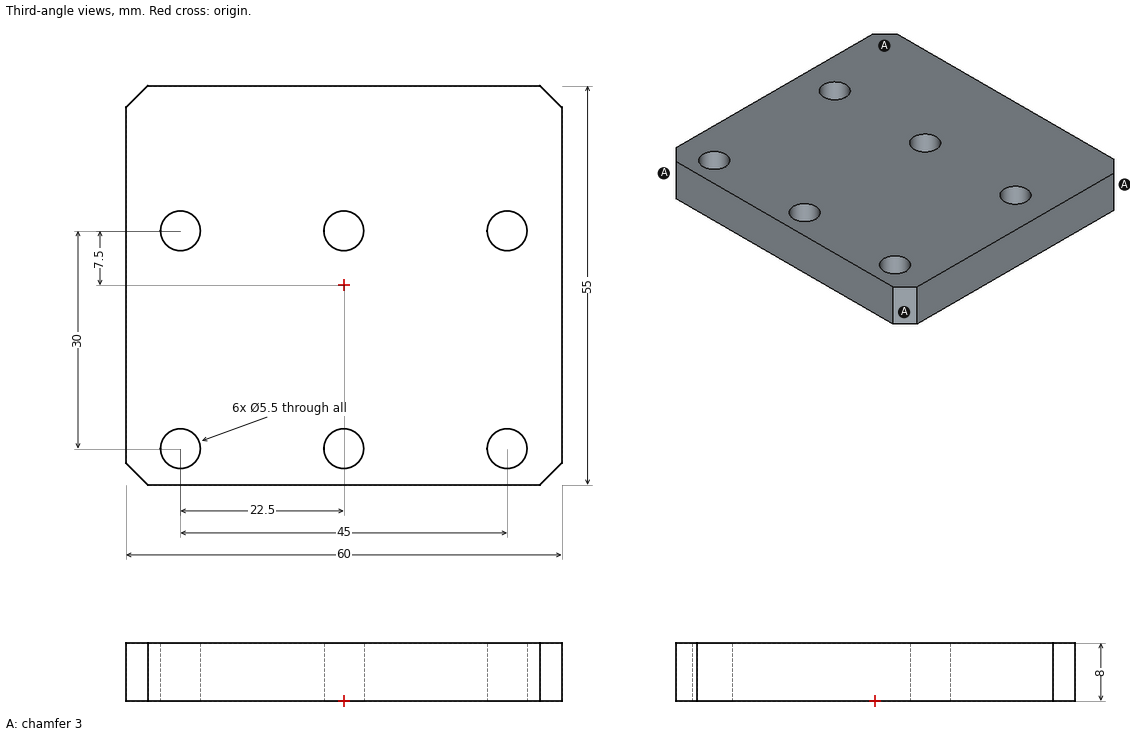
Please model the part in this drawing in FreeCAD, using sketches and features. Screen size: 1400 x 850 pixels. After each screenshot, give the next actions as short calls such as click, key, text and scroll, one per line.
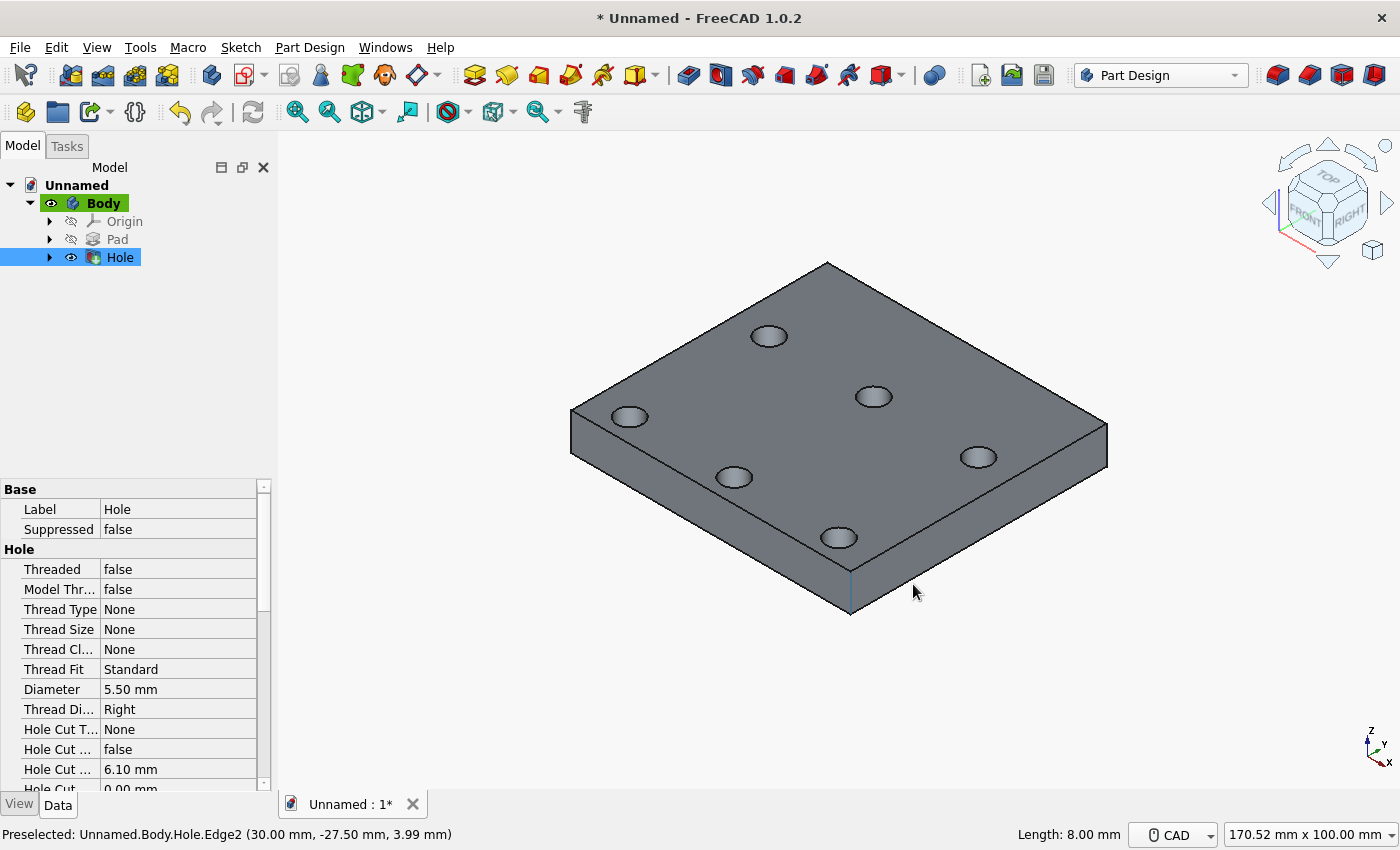
key(2)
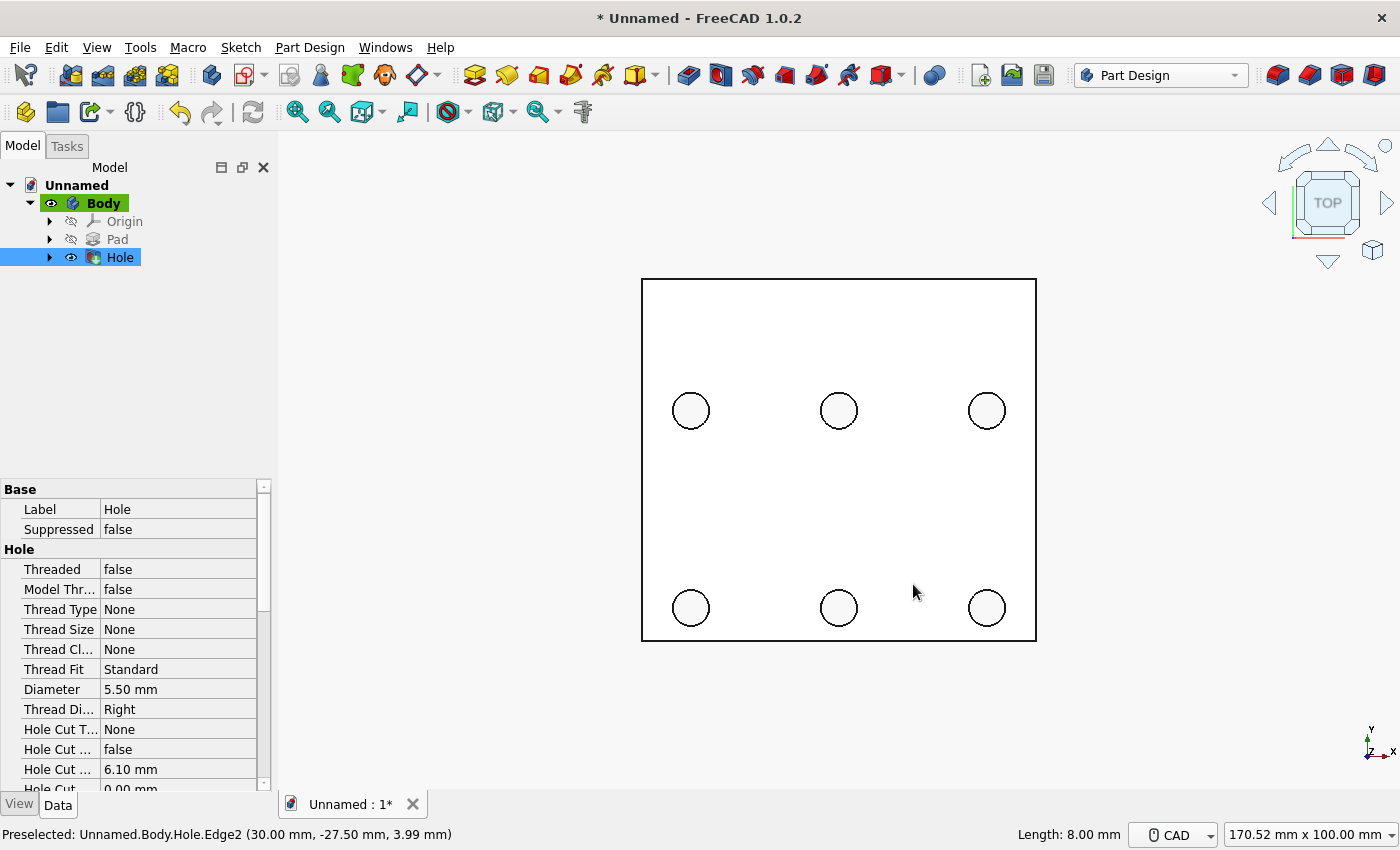
key(1)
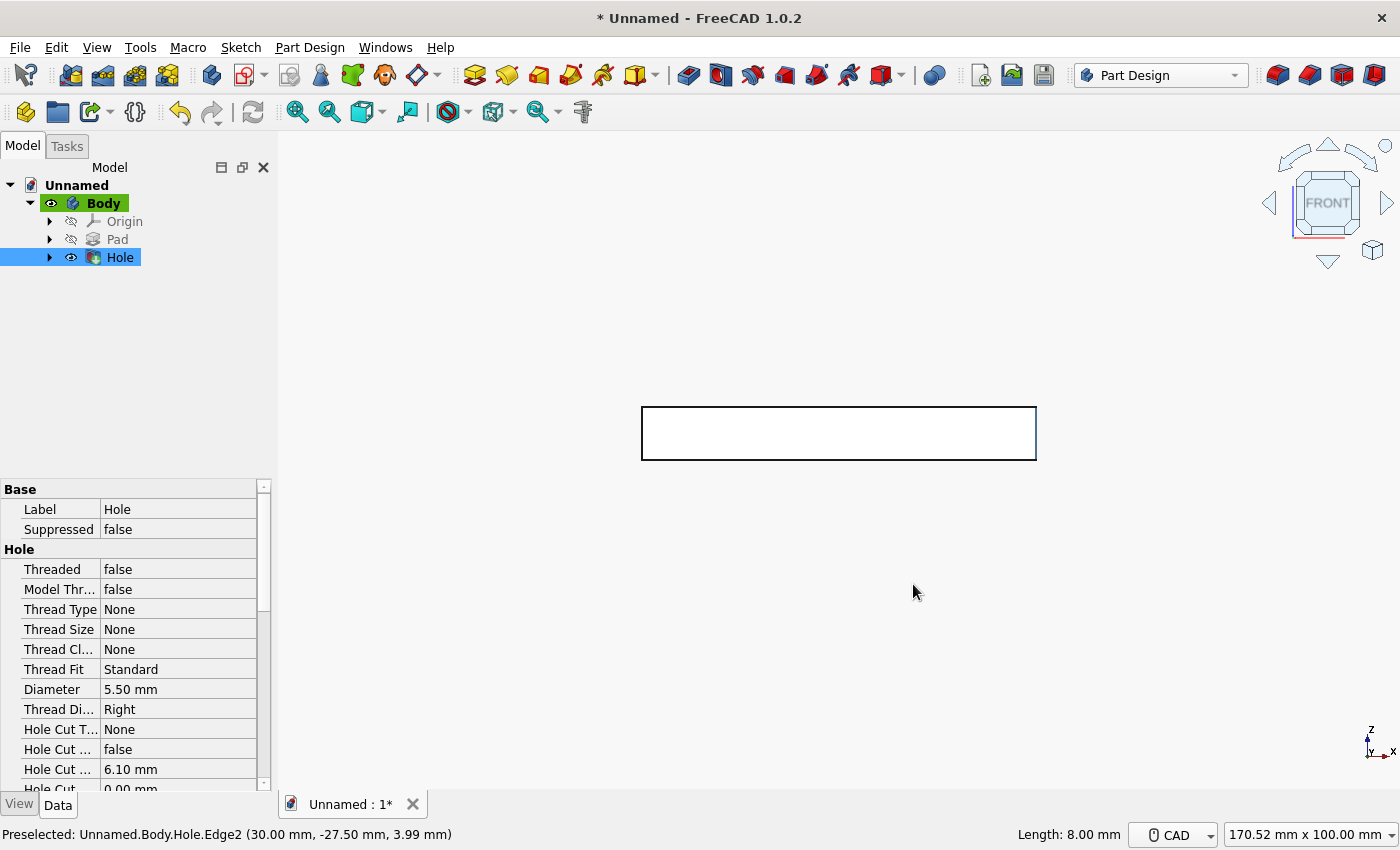
click(298, 112)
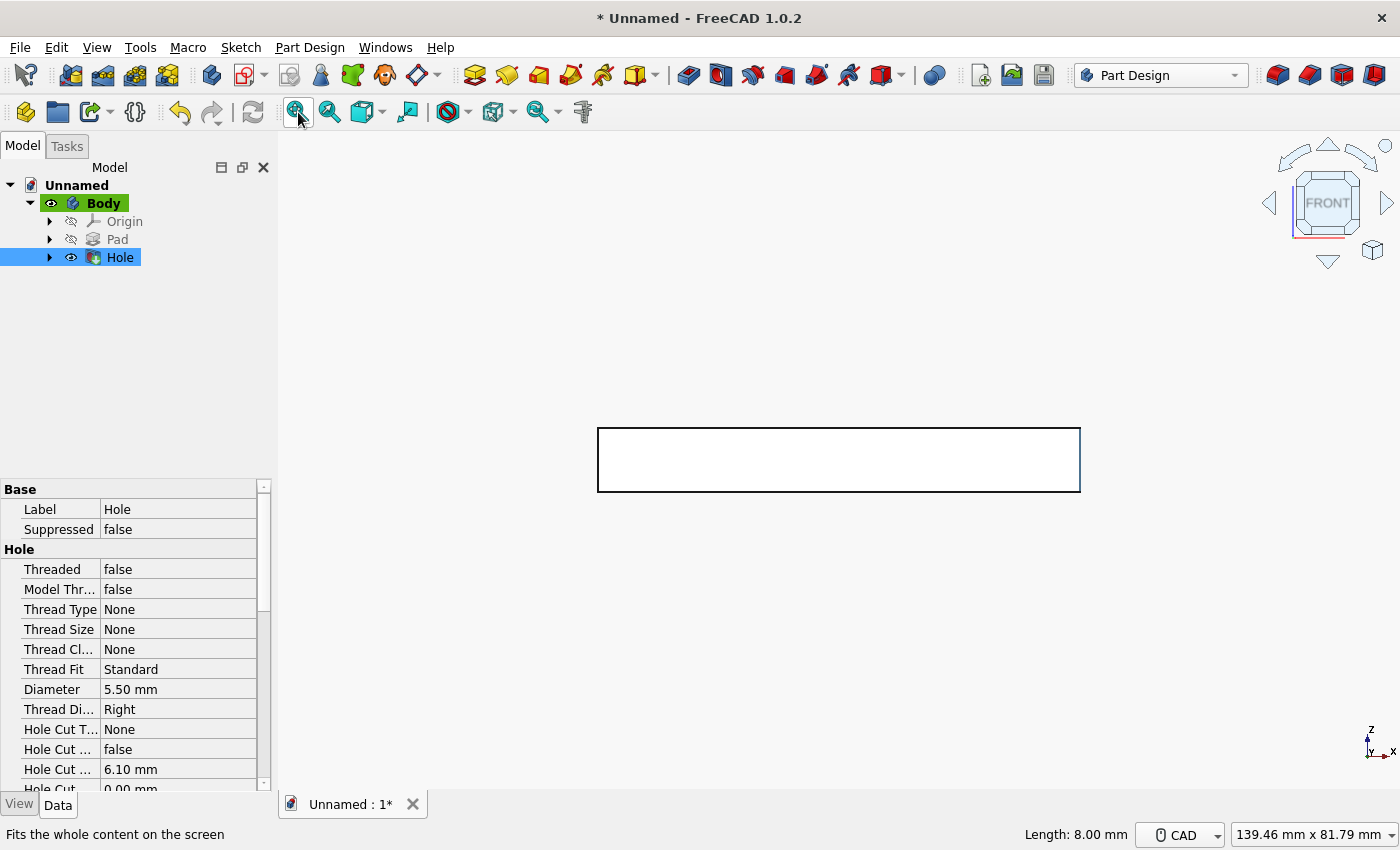
click(598, 459, ctrl)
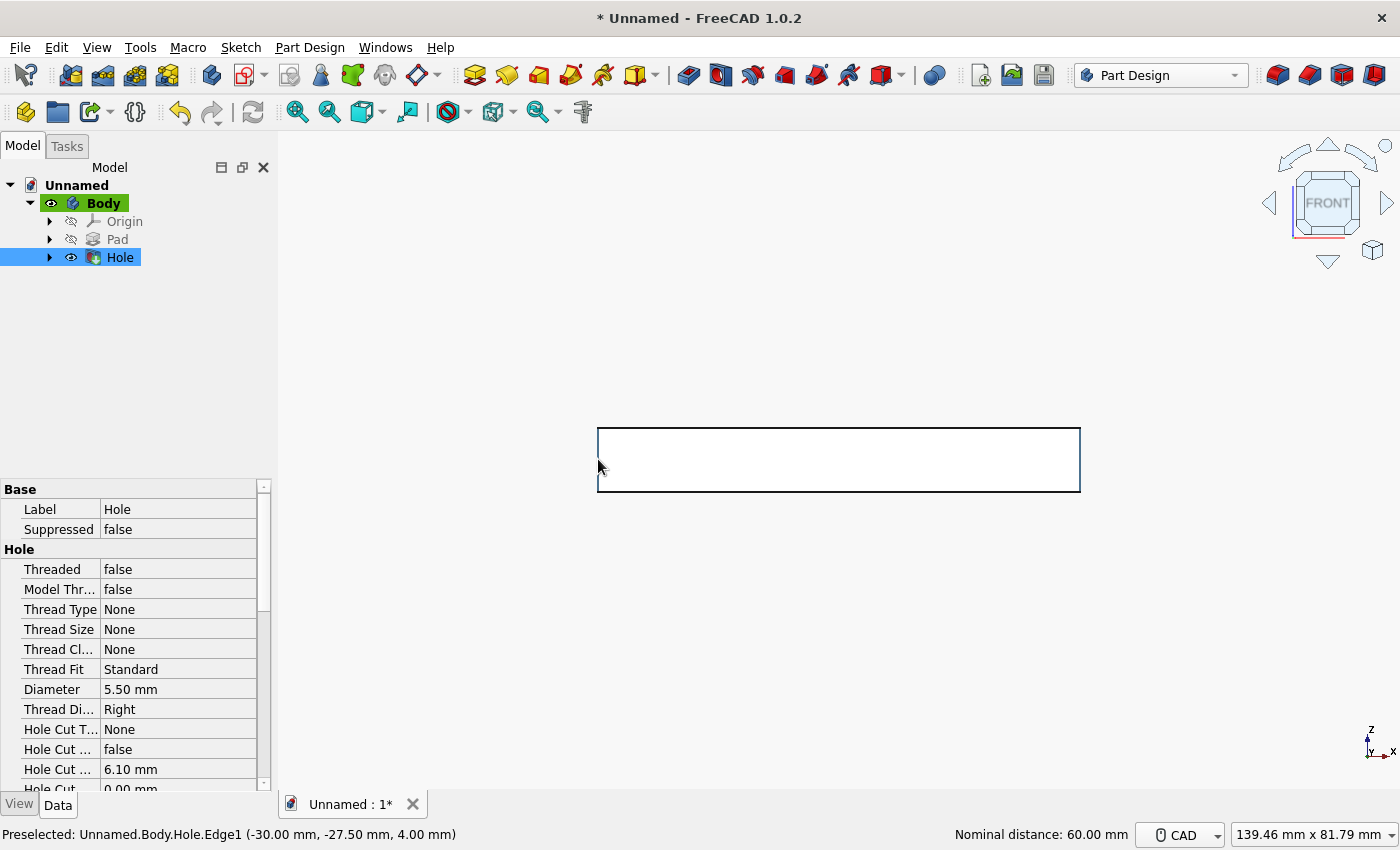
key(3)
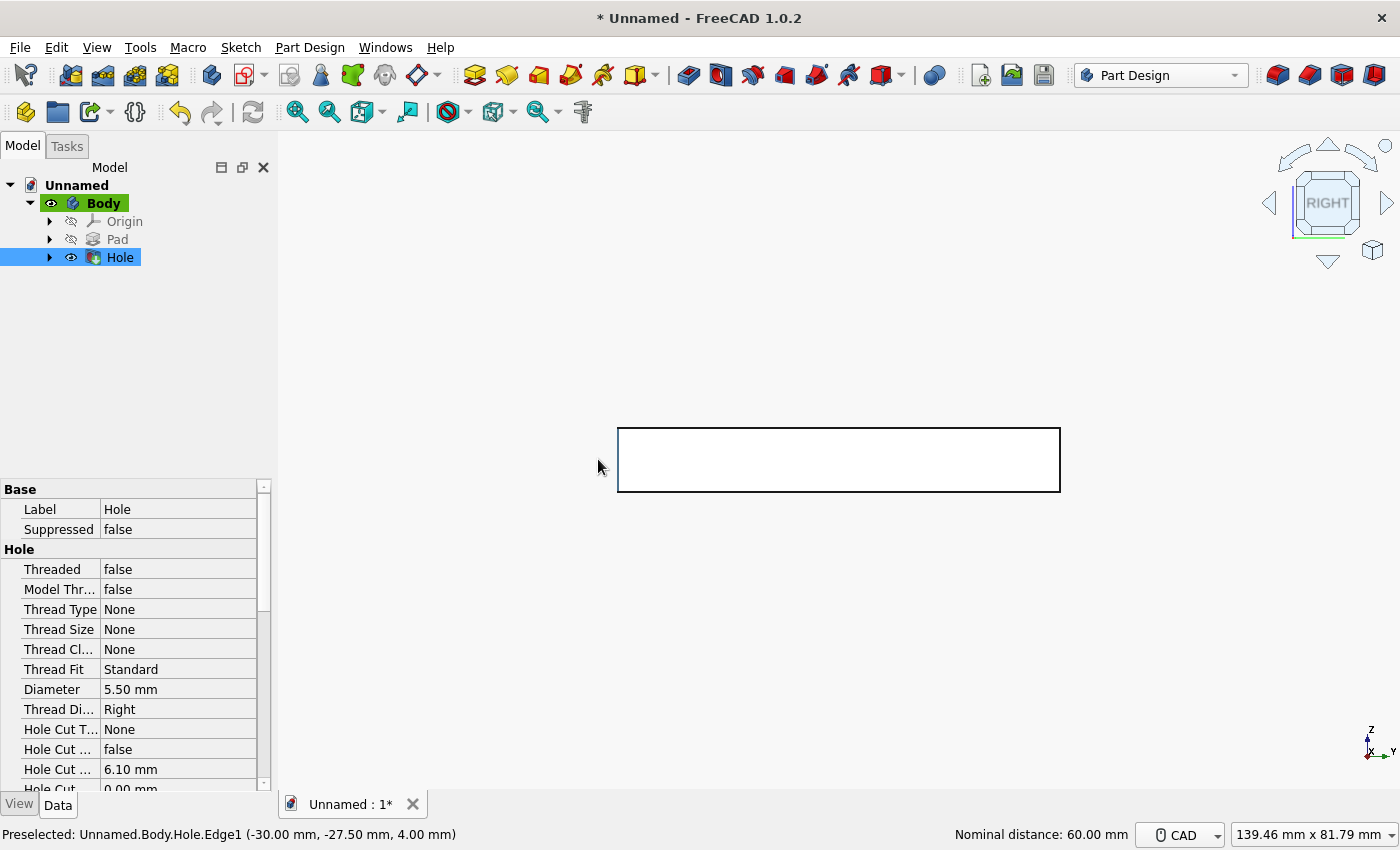
click(298, 112)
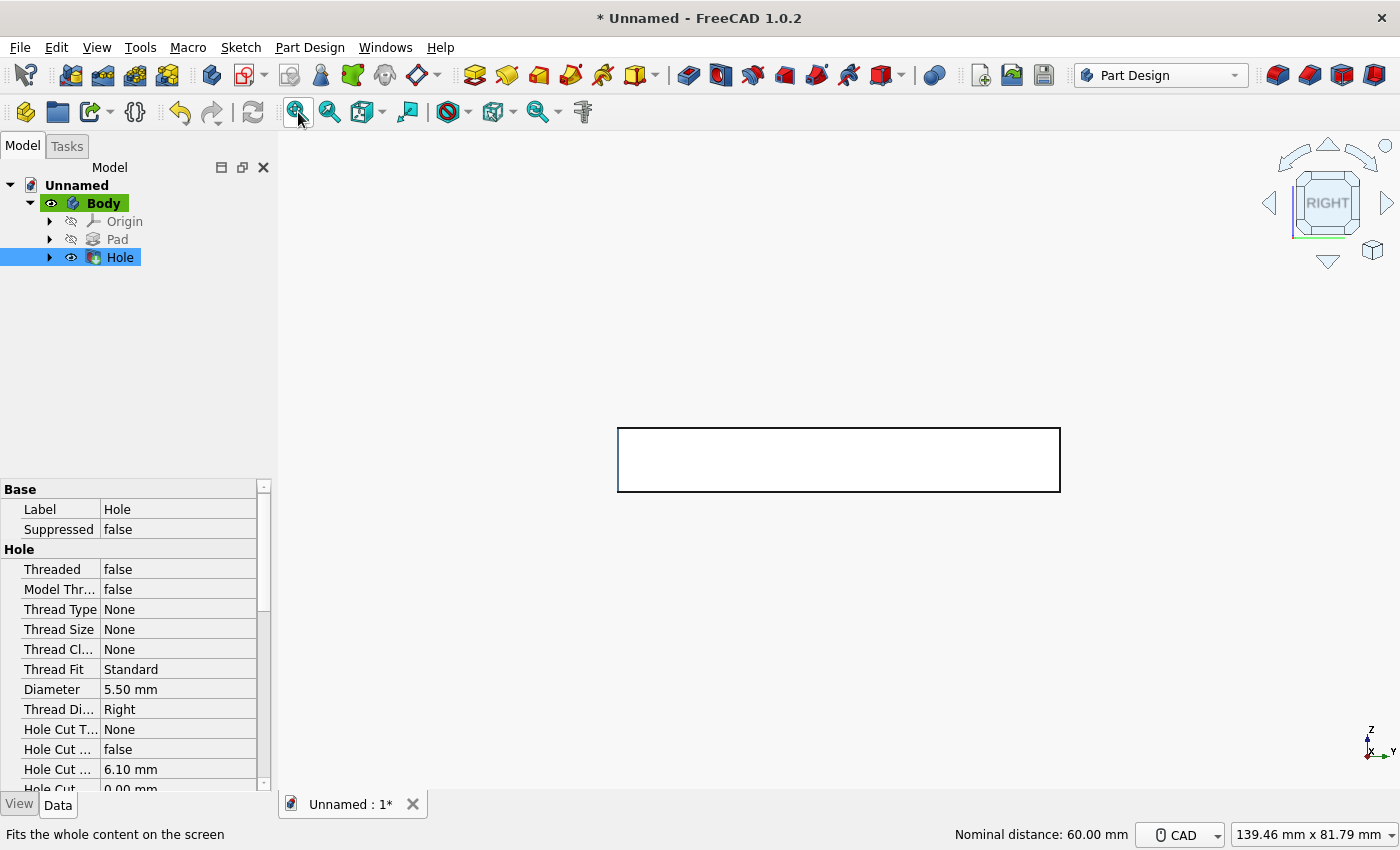
click(1060, 459, ctrl)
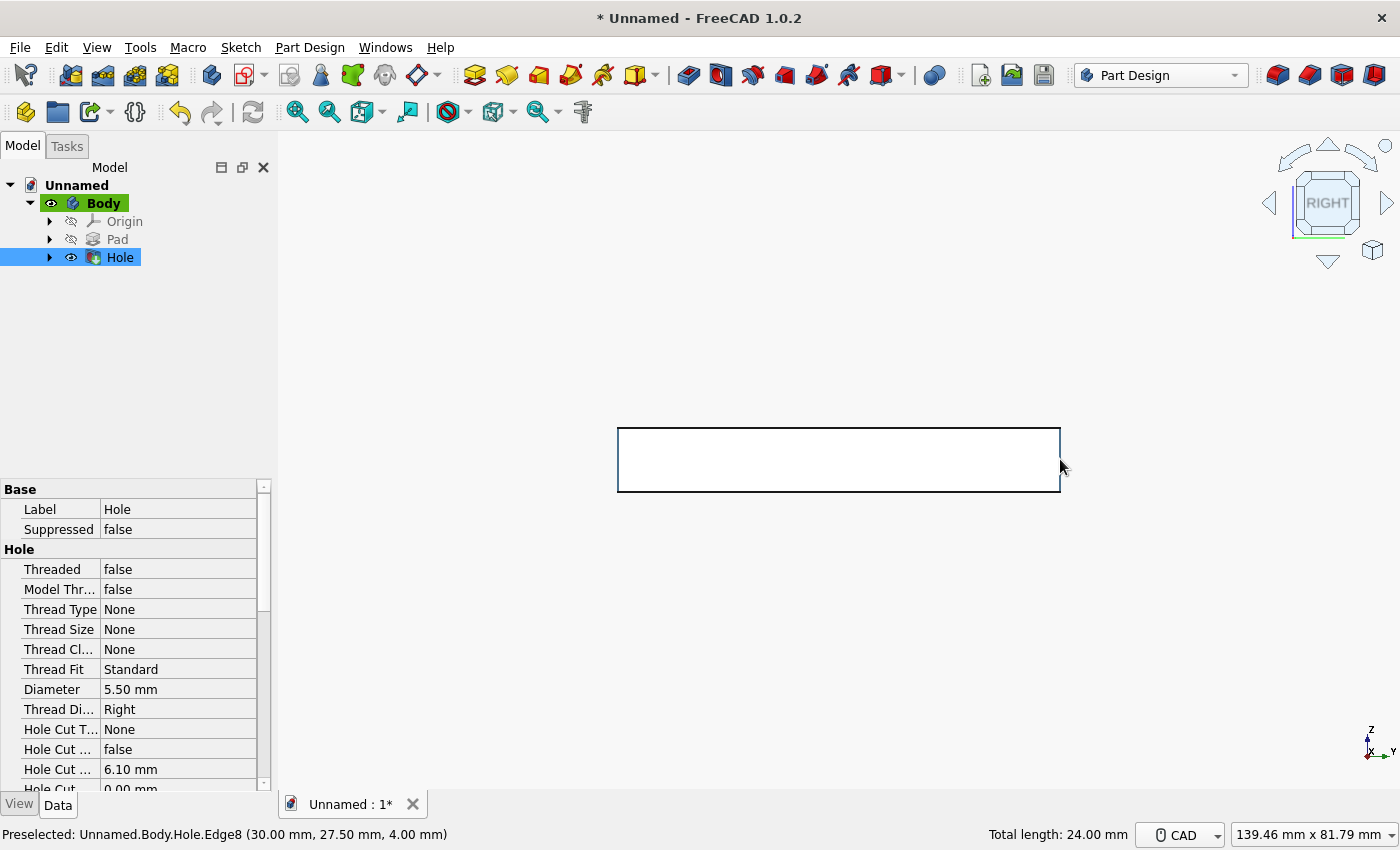
key(5)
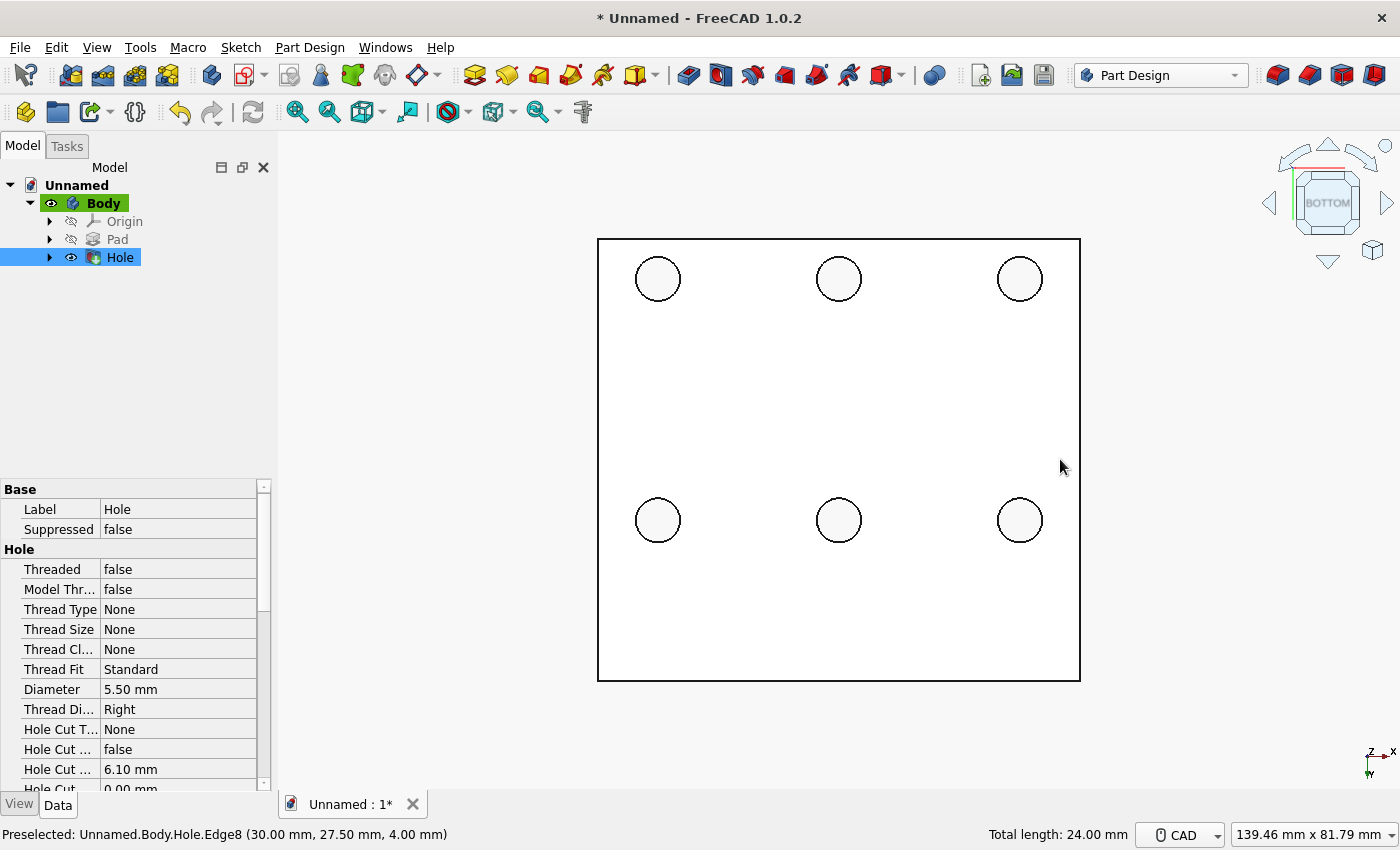
key(4)